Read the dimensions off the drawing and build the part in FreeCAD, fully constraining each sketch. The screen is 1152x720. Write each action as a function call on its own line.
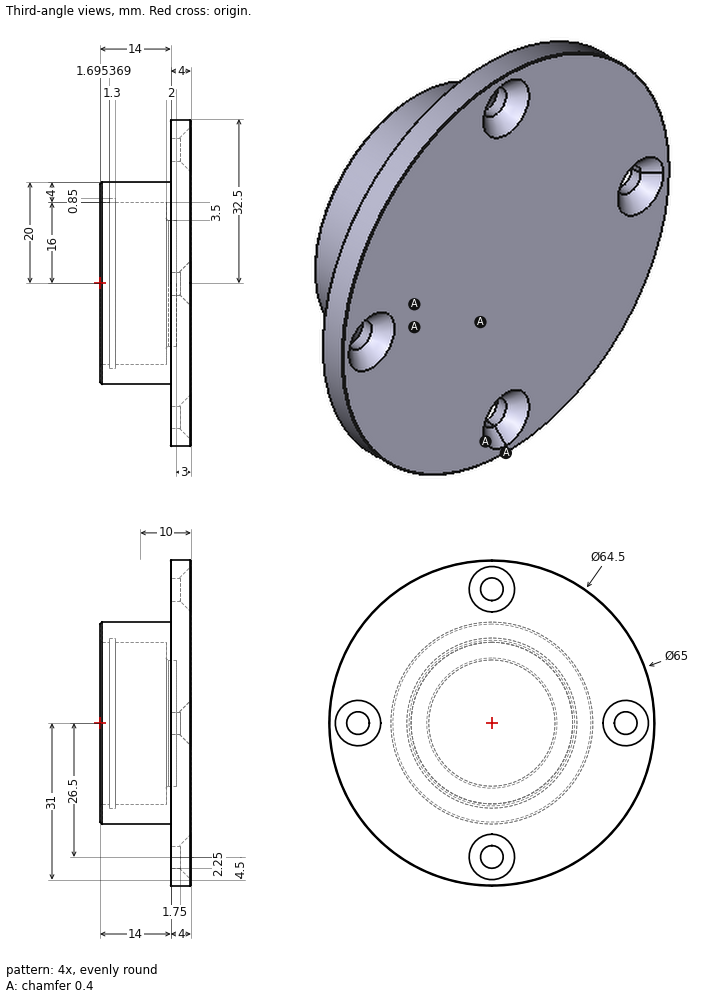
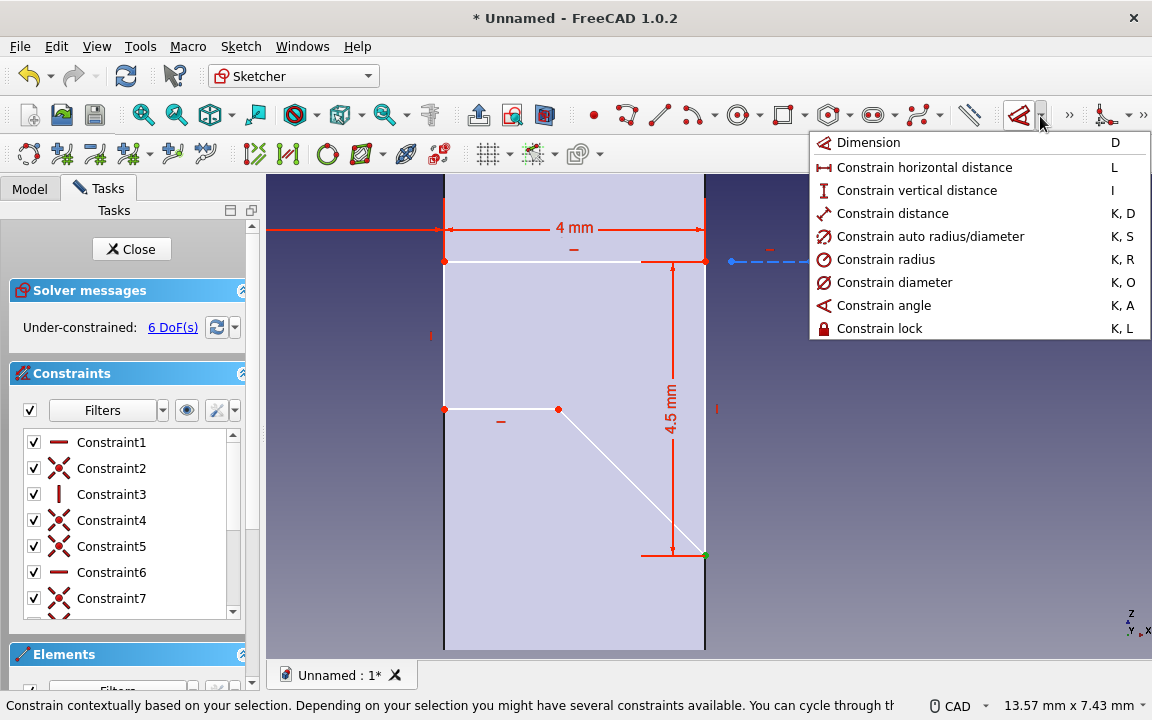
click(980, 190)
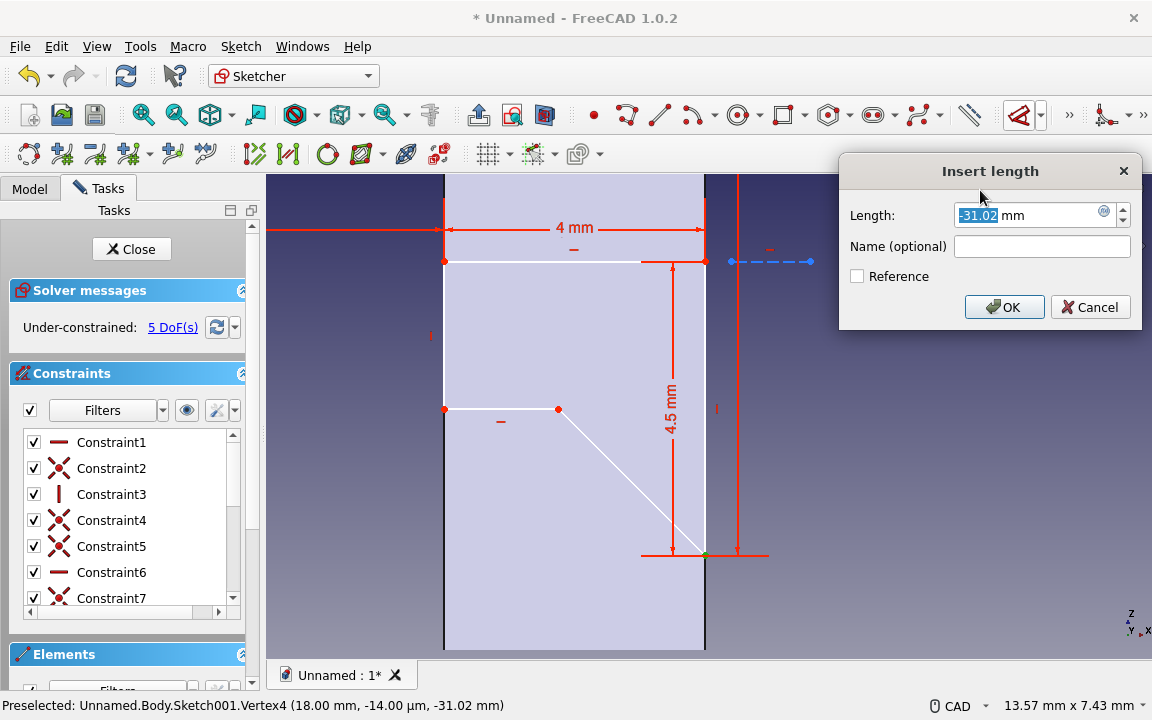
text(-31)
key(Return)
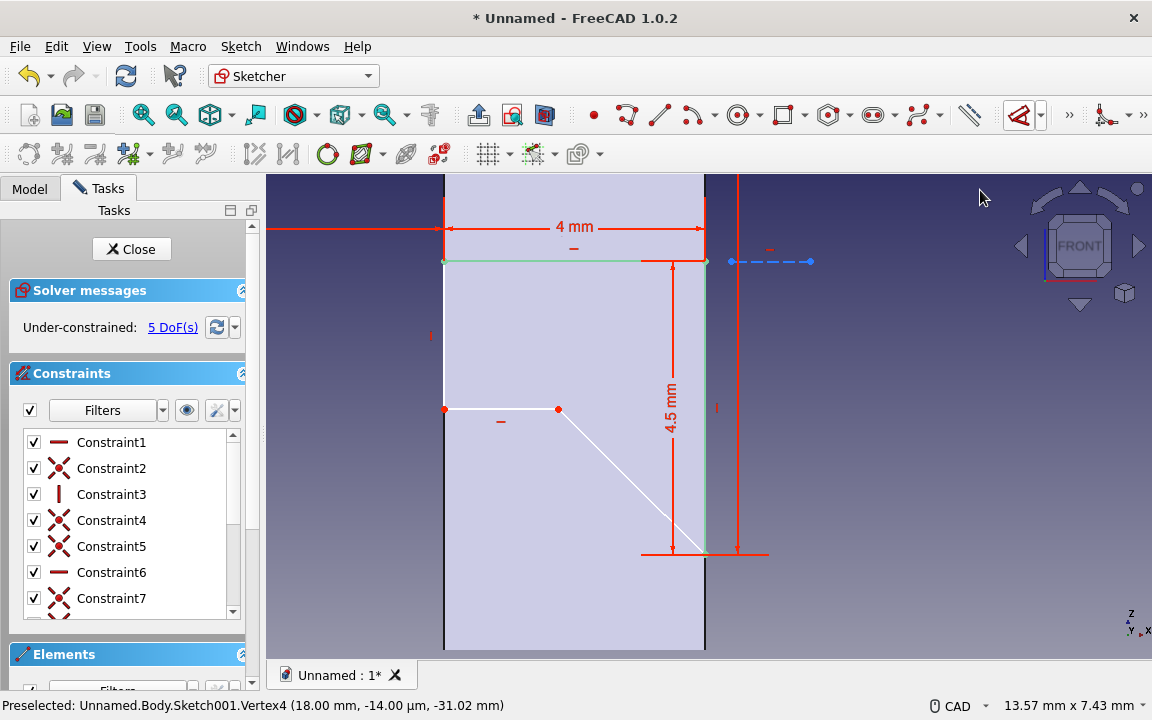
click(524, 409)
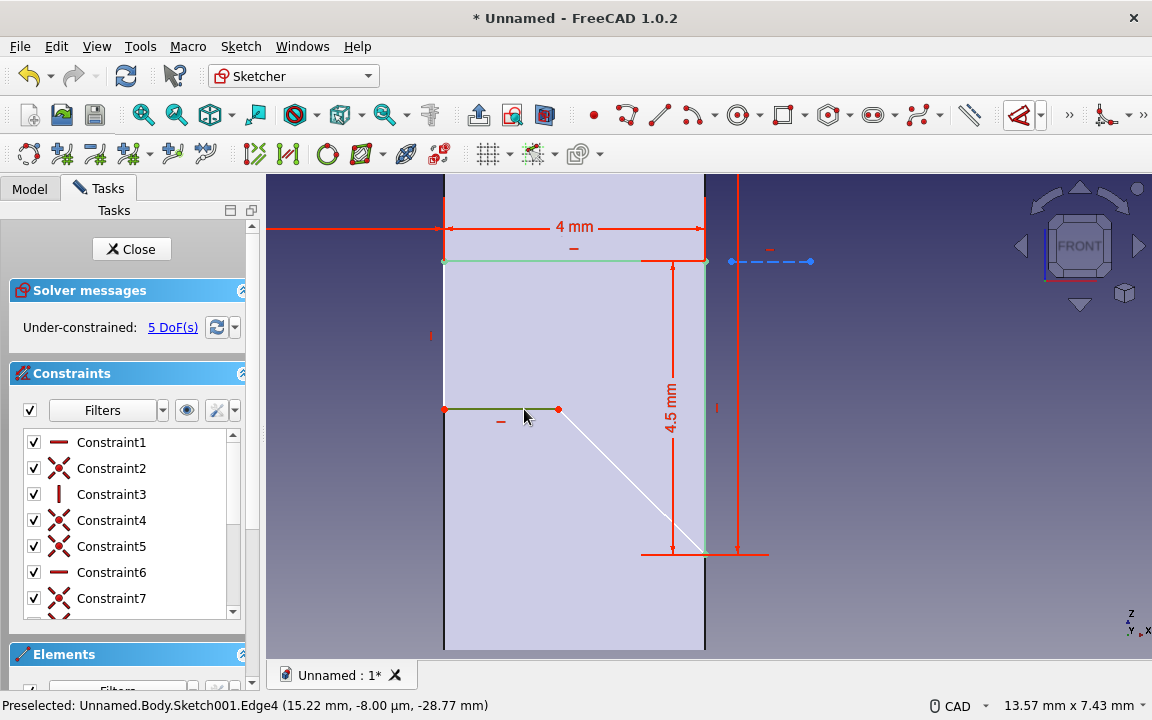
key(l)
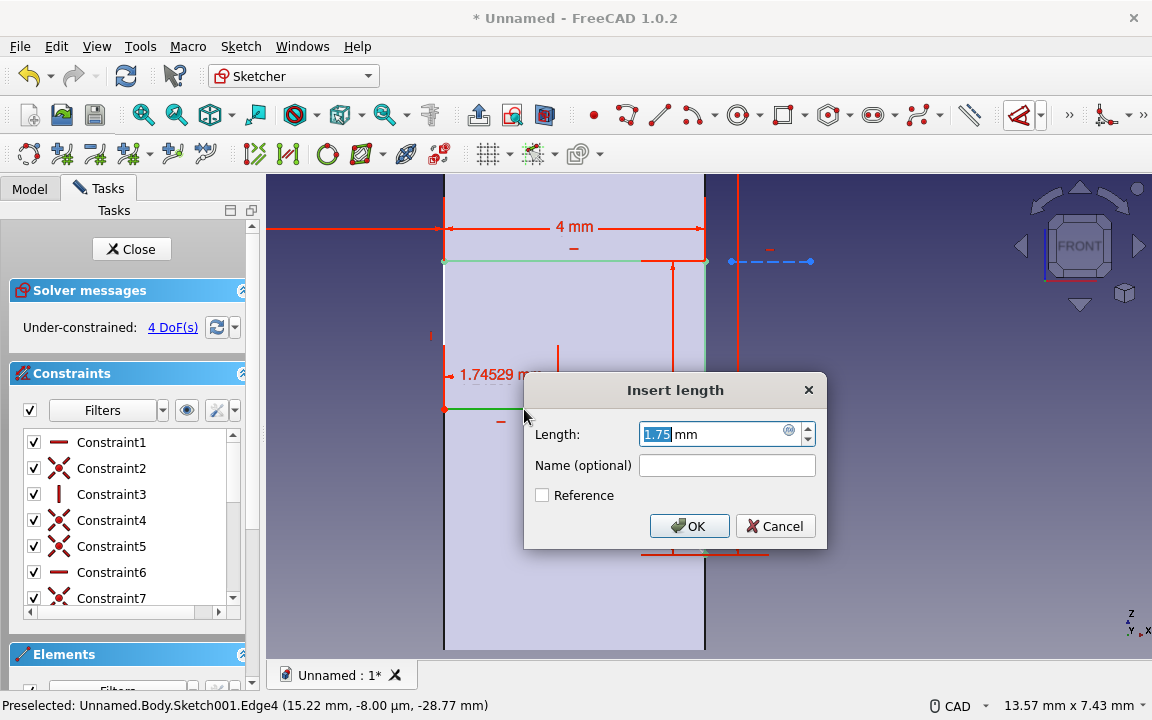
text(1.75)
key(Return)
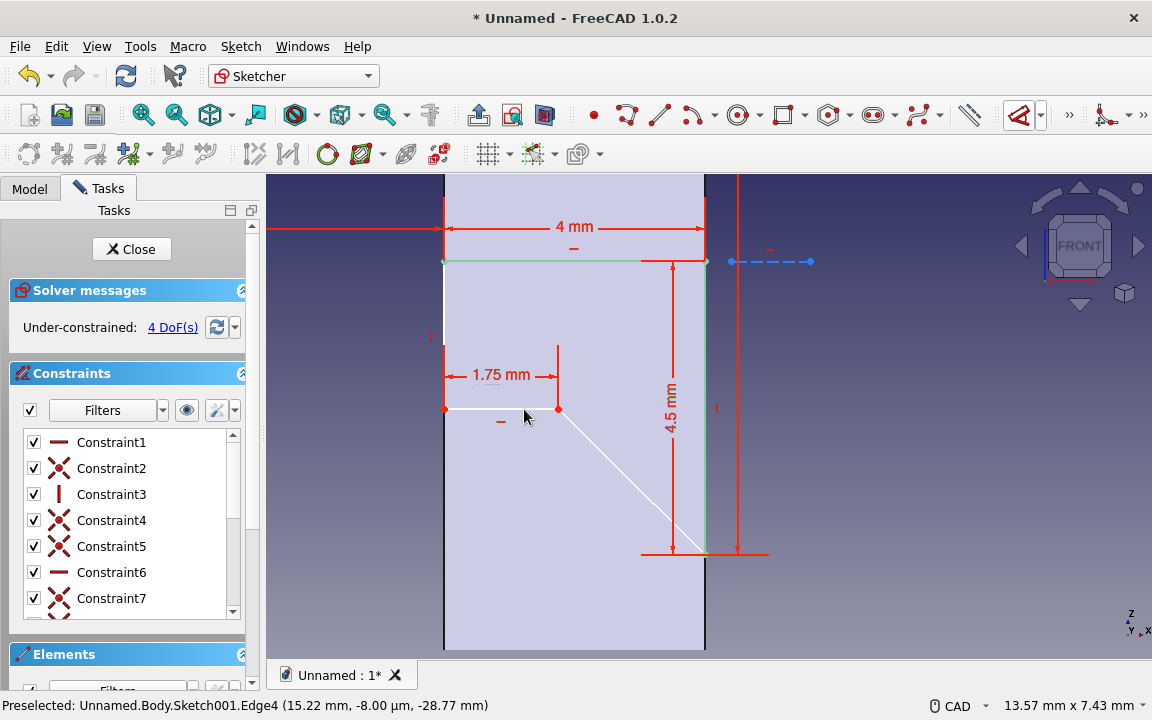
click(444, 365)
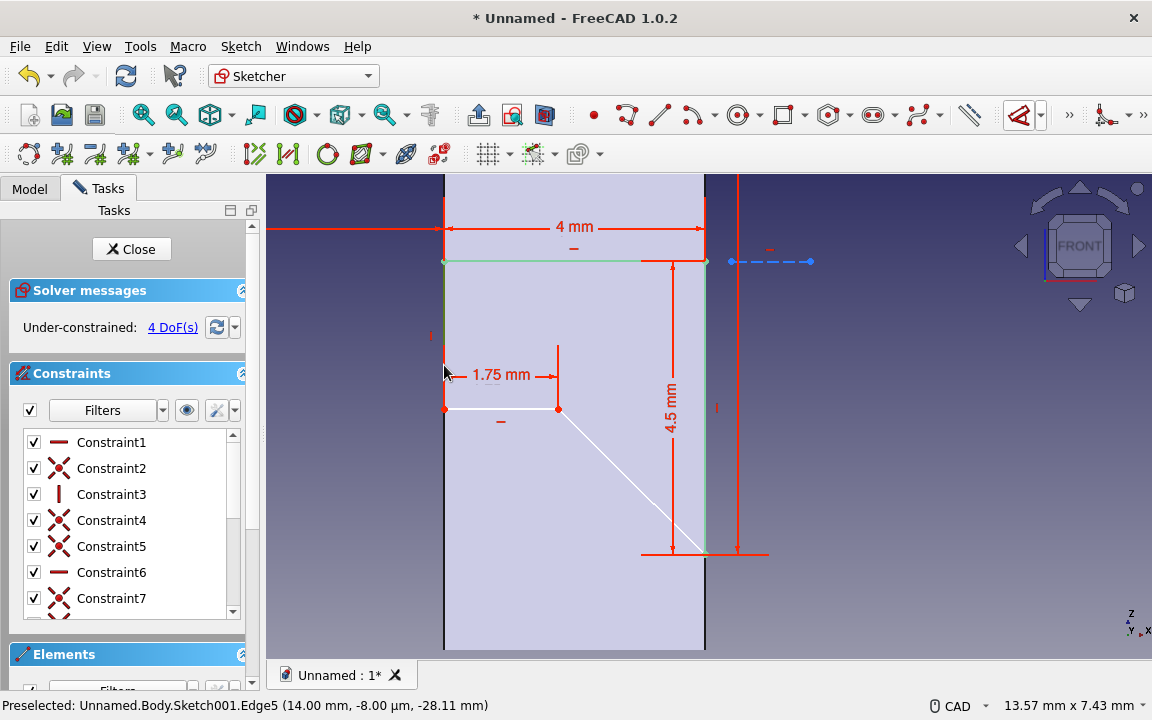
key(i)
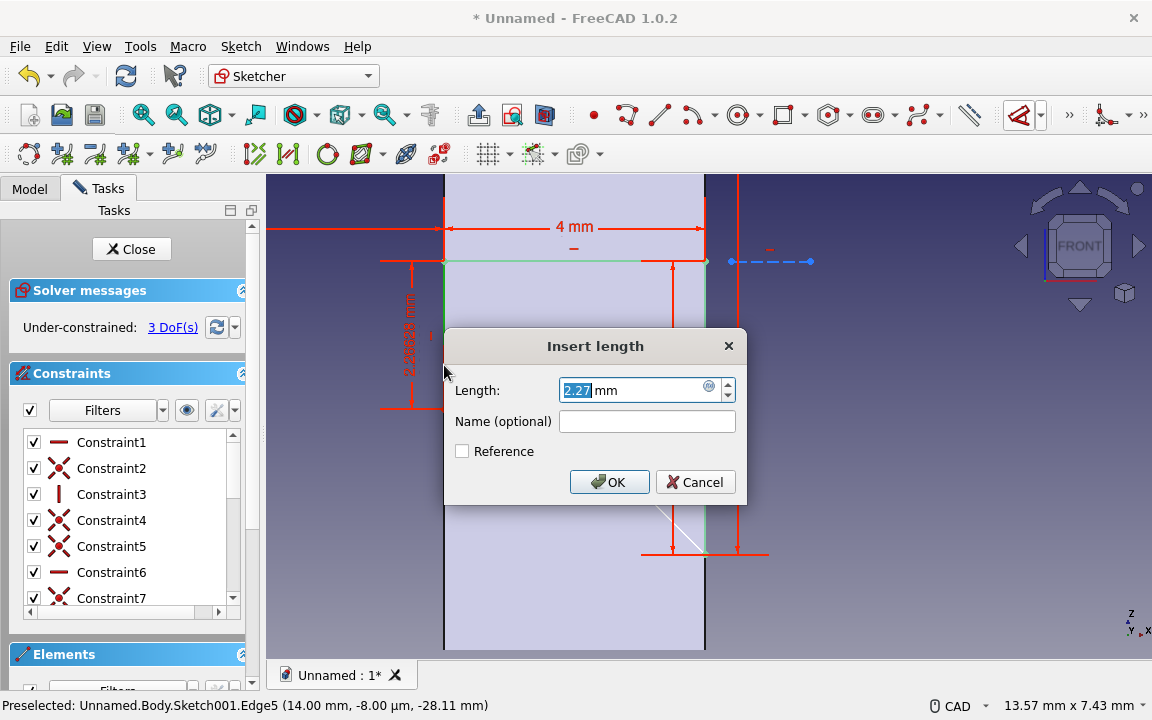
text(2.25)
key(Return)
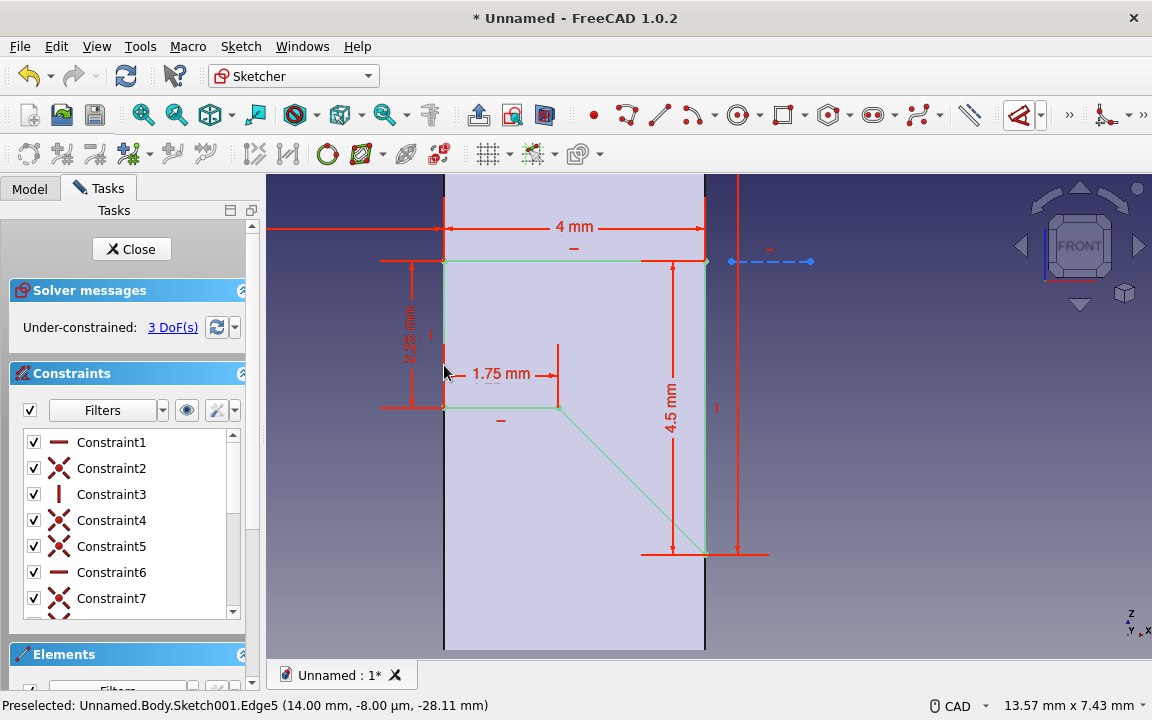
click(731, 262)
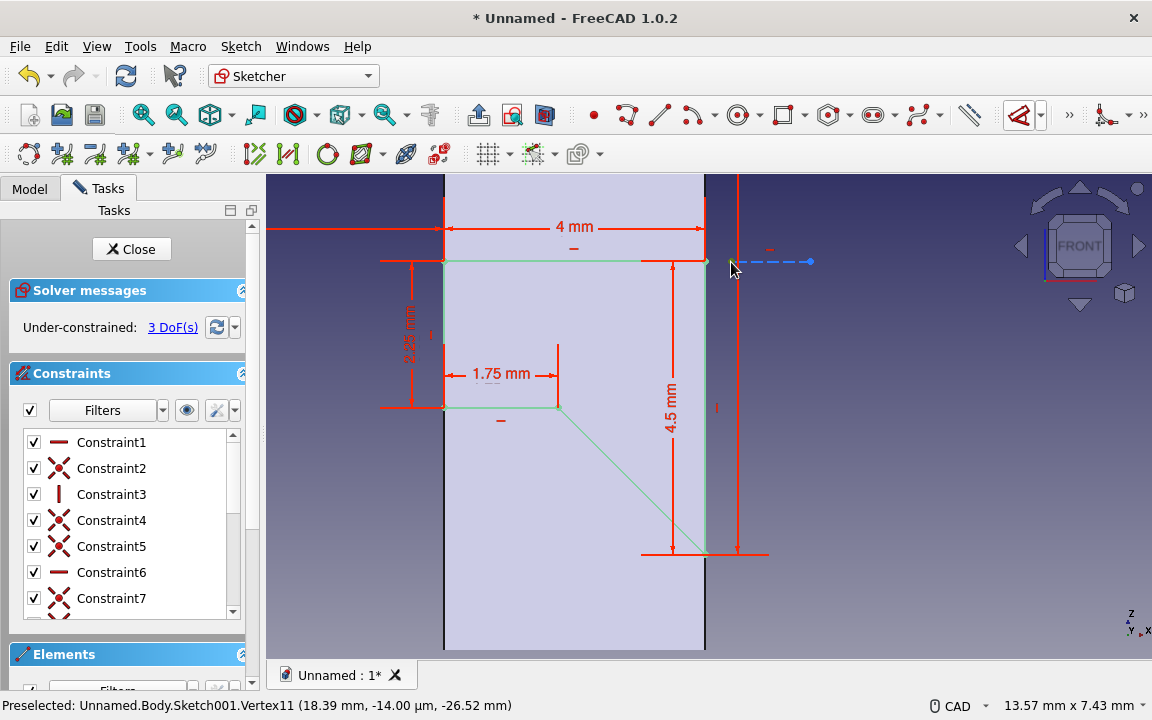
click(1040, 116)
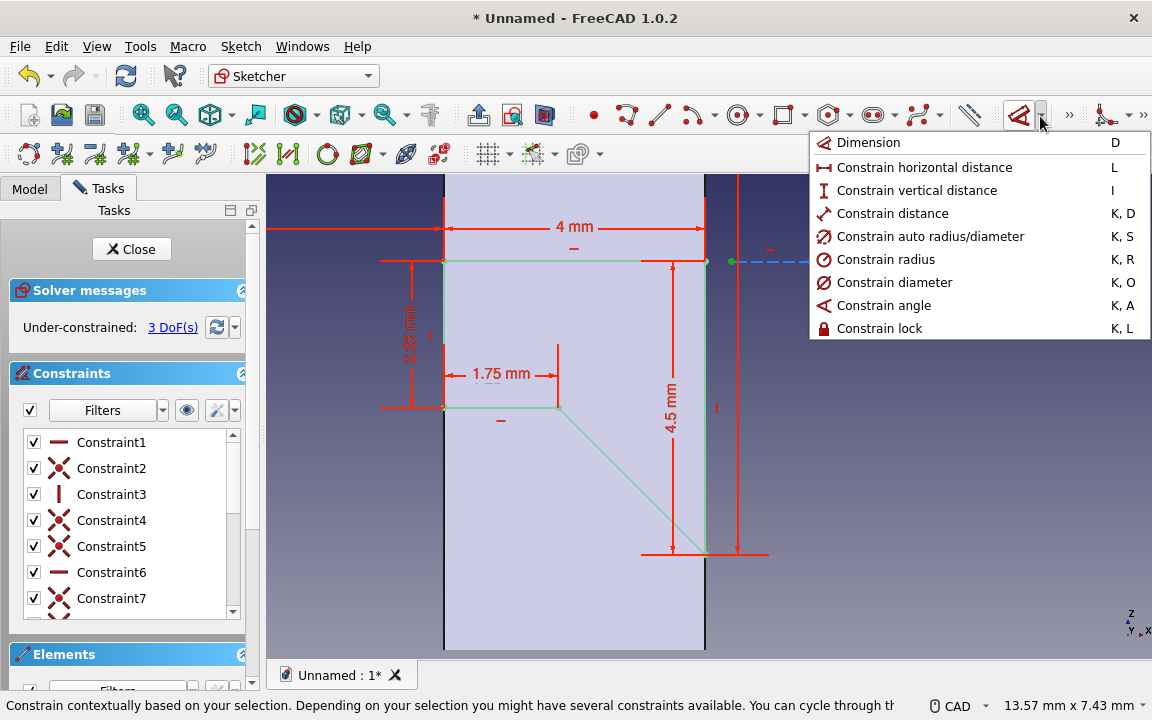
click(980, 190)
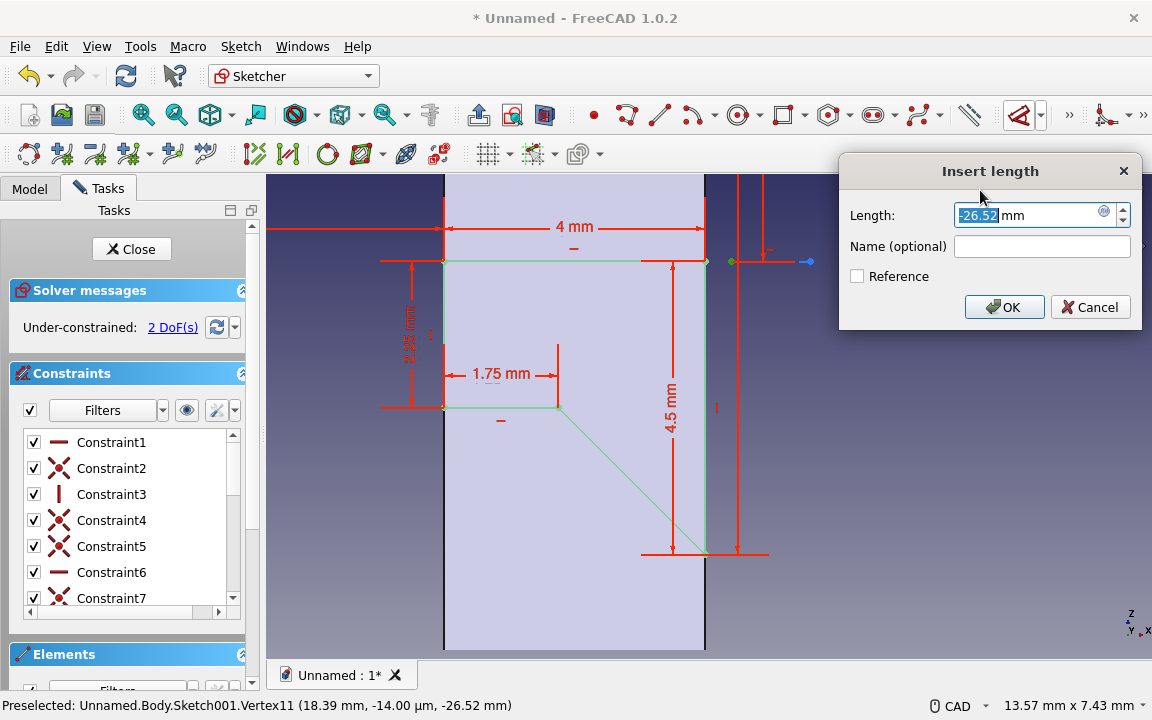
text(-26.5)
key(Return)